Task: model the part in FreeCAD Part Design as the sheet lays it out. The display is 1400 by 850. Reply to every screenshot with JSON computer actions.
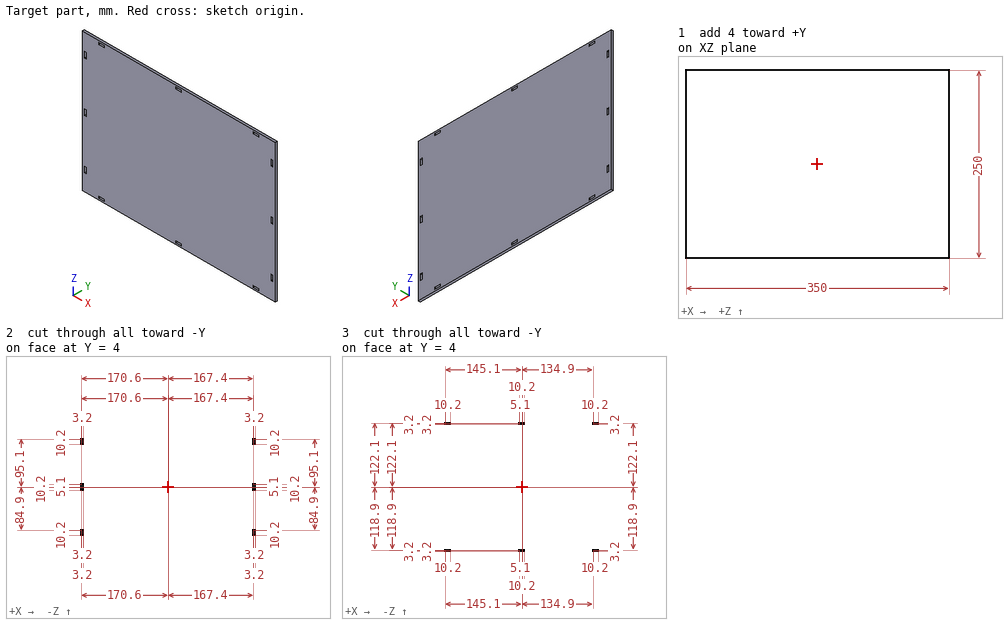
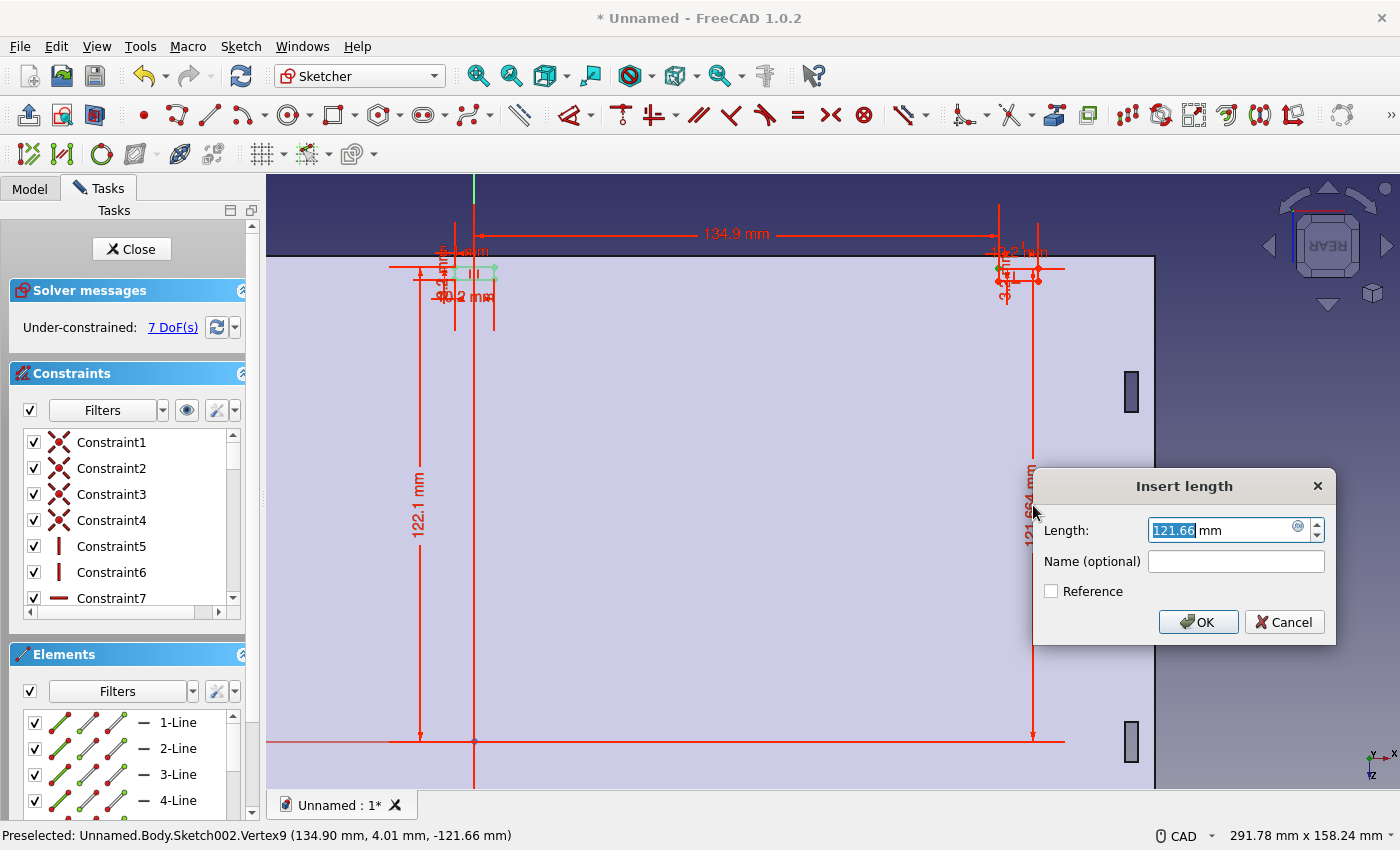
{"action": "type", "text": "122.1"}
{"action": "key", "text": "Return"}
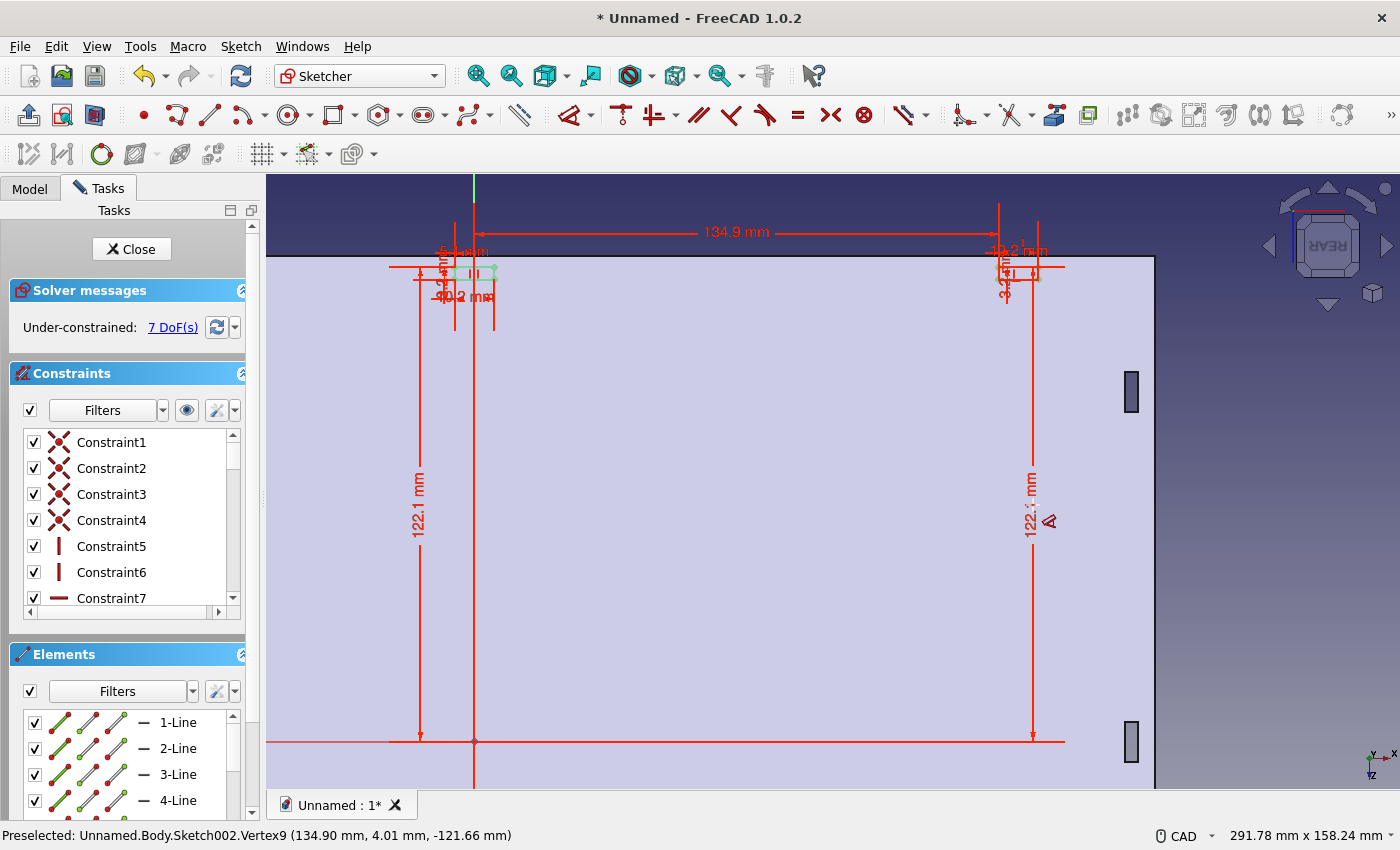
{"action": "scroll", "coordinate": [1001, 269], "scroll_direction": "down", "scroll_amount": 4}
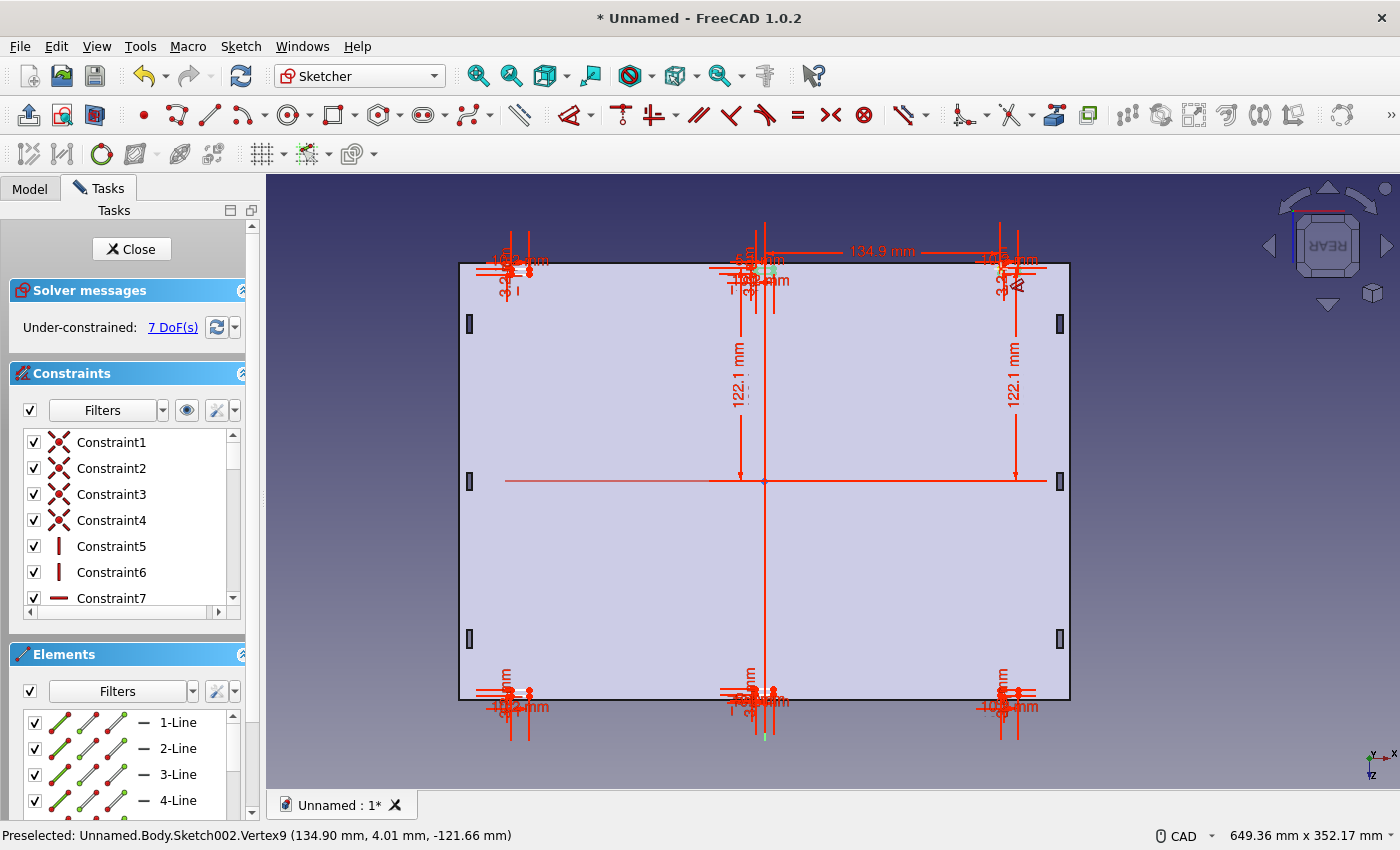
{"action": "scroll", "coordinate": [511, 269], "scroll_direction": "up", "scroll_amount": 4}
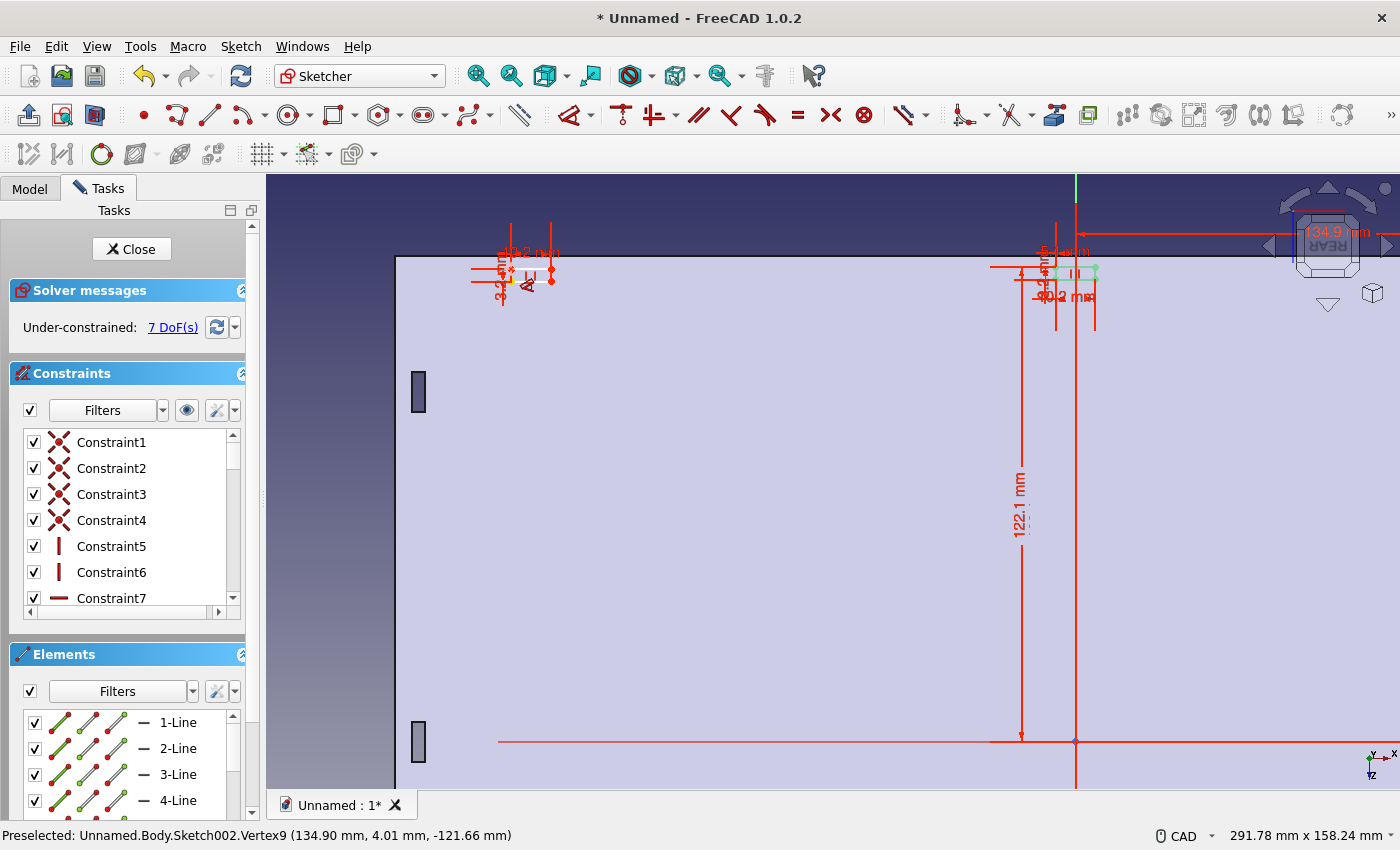
{"action": "left_click", "coordinate": [511, 269]}
{"action": "left_click", "coordinate": [793, 235]}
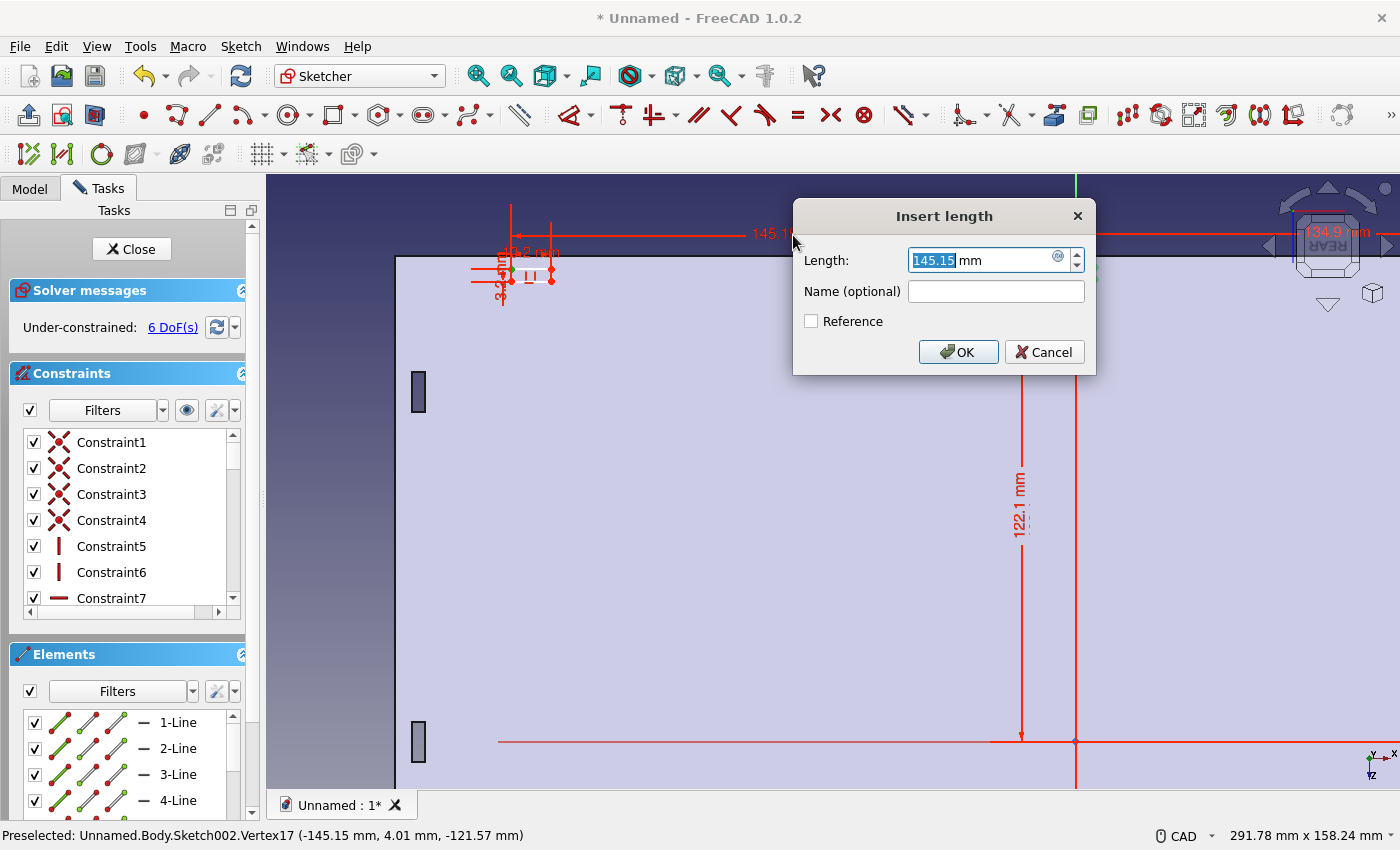
{"action": "type", "text": "145.1"}
{"action": "key", "text": "Return"}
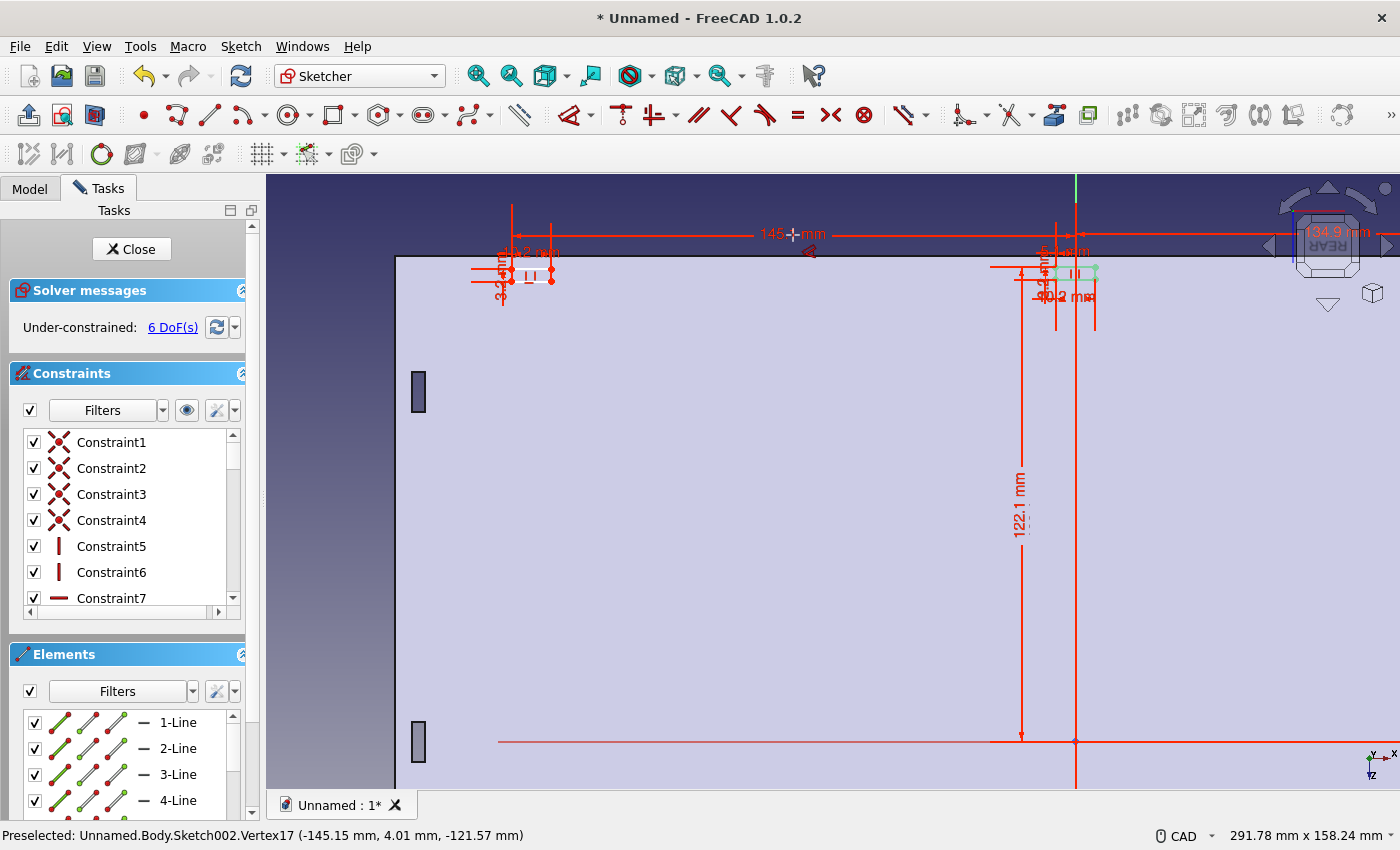
{"action": "left_click", "coordinate": [512, 269]}
{"action": "left_click", "coordinate": [478, 505]}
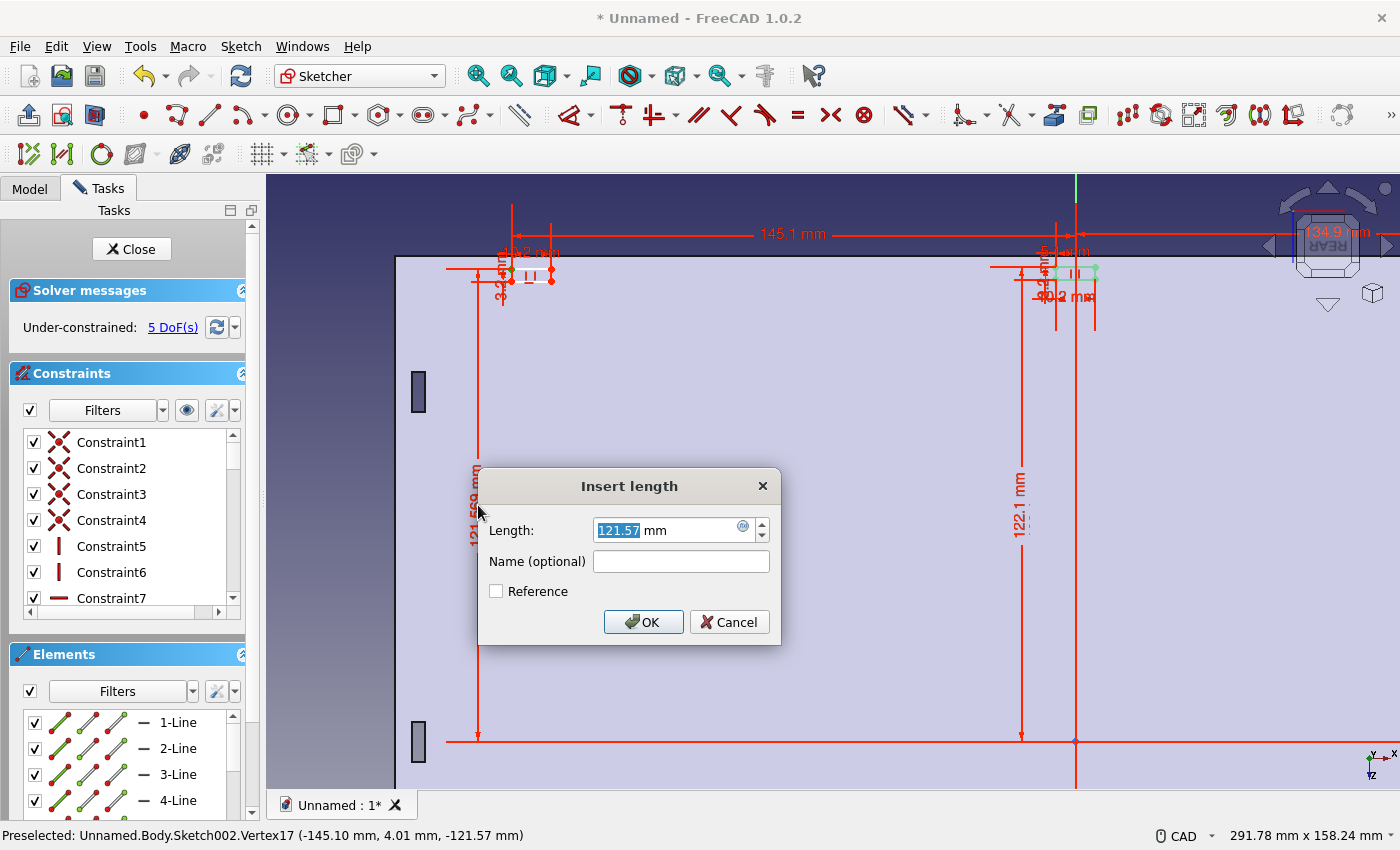
{"action": "type", "text": "122.1"}
{"action": "key", "text": "Return"}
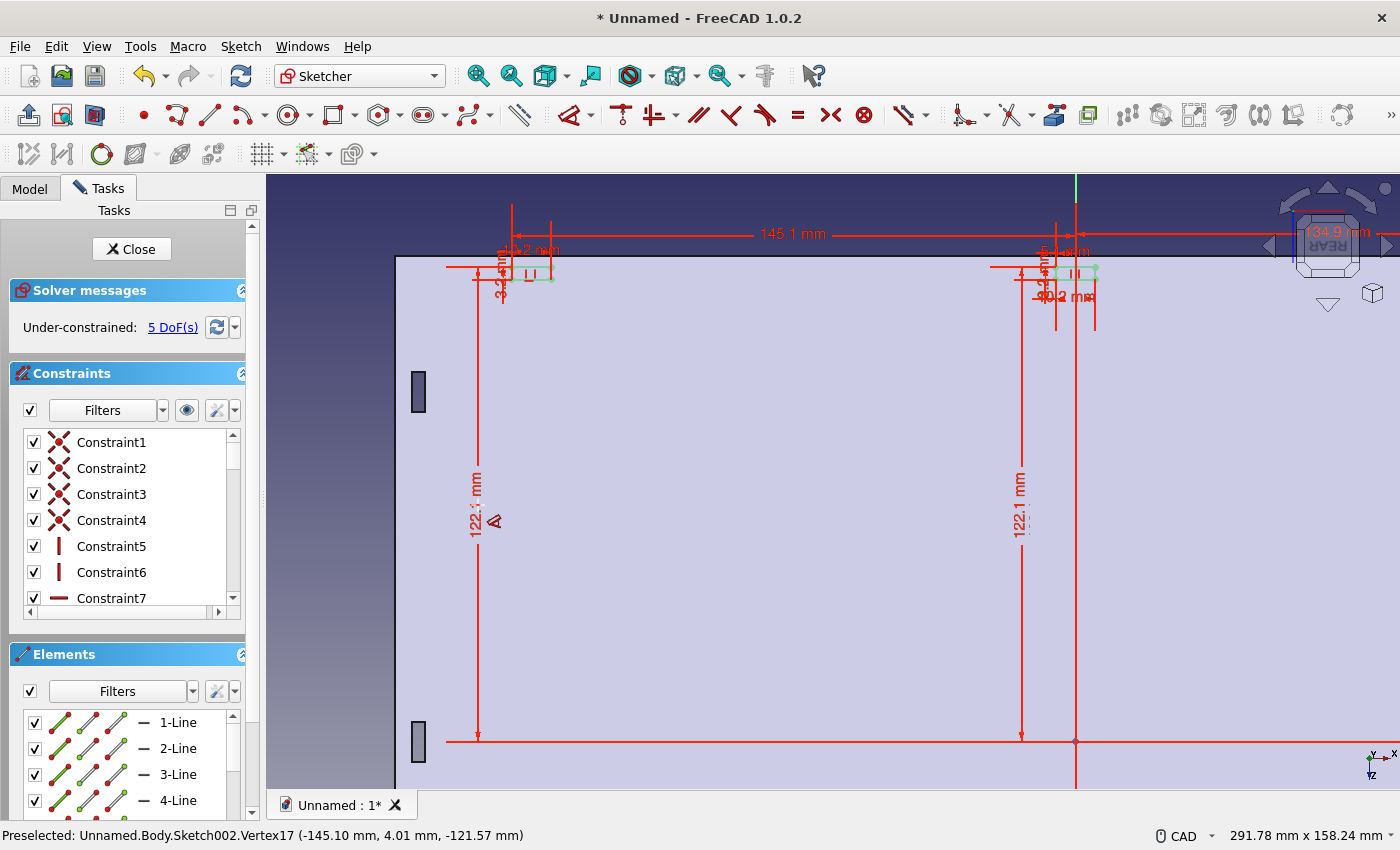
{"action": "scroll", "coordinate": [511, 269], "scroll_direction": "down", "scroll_amount": 4}